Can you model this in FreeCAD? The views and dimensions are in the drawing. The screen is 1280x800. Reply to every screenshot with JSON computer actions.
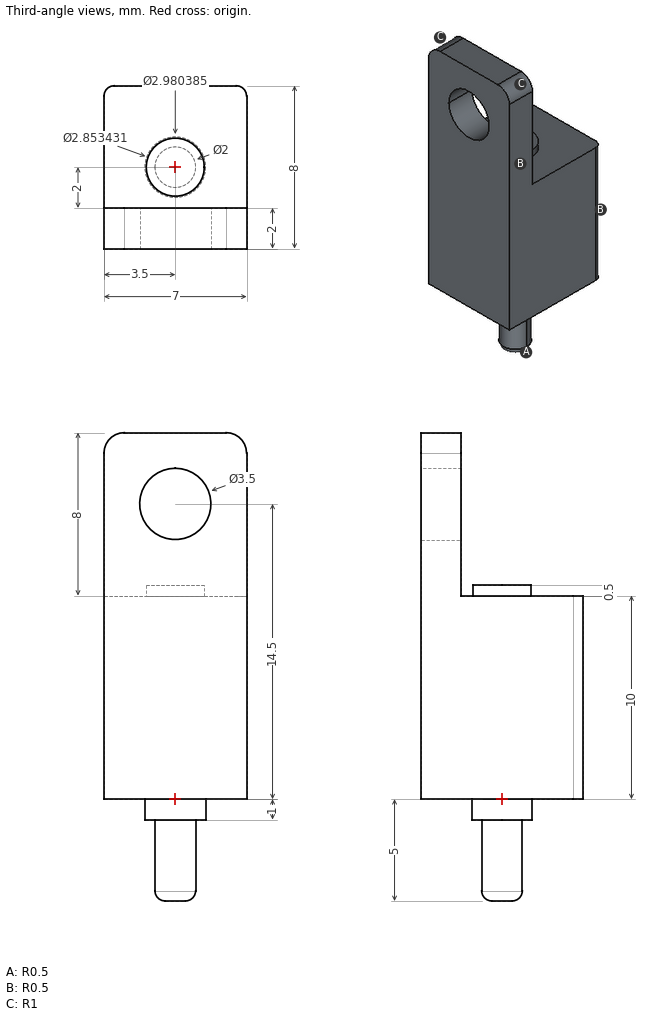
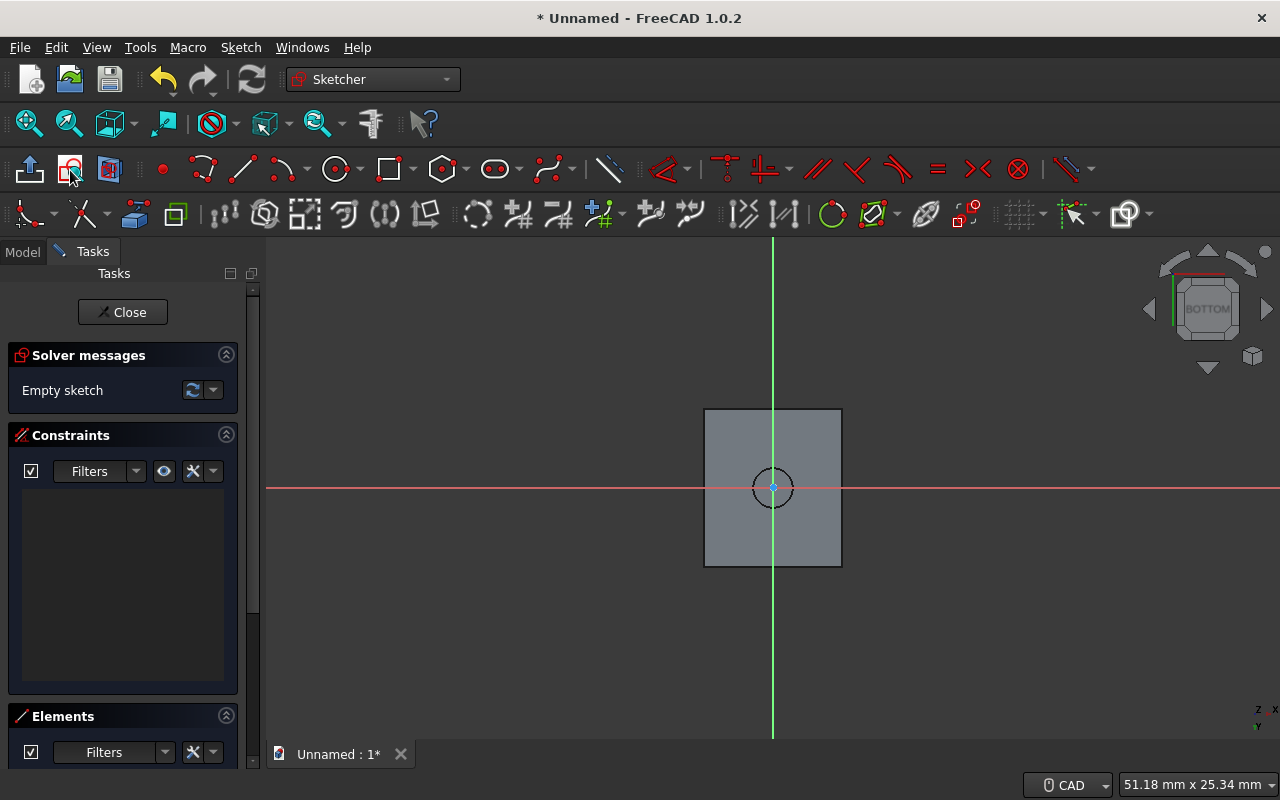
{"action": "scroll", "coordinate": [790, 488], "scroll_direction": "up", "scroll_amount": 8}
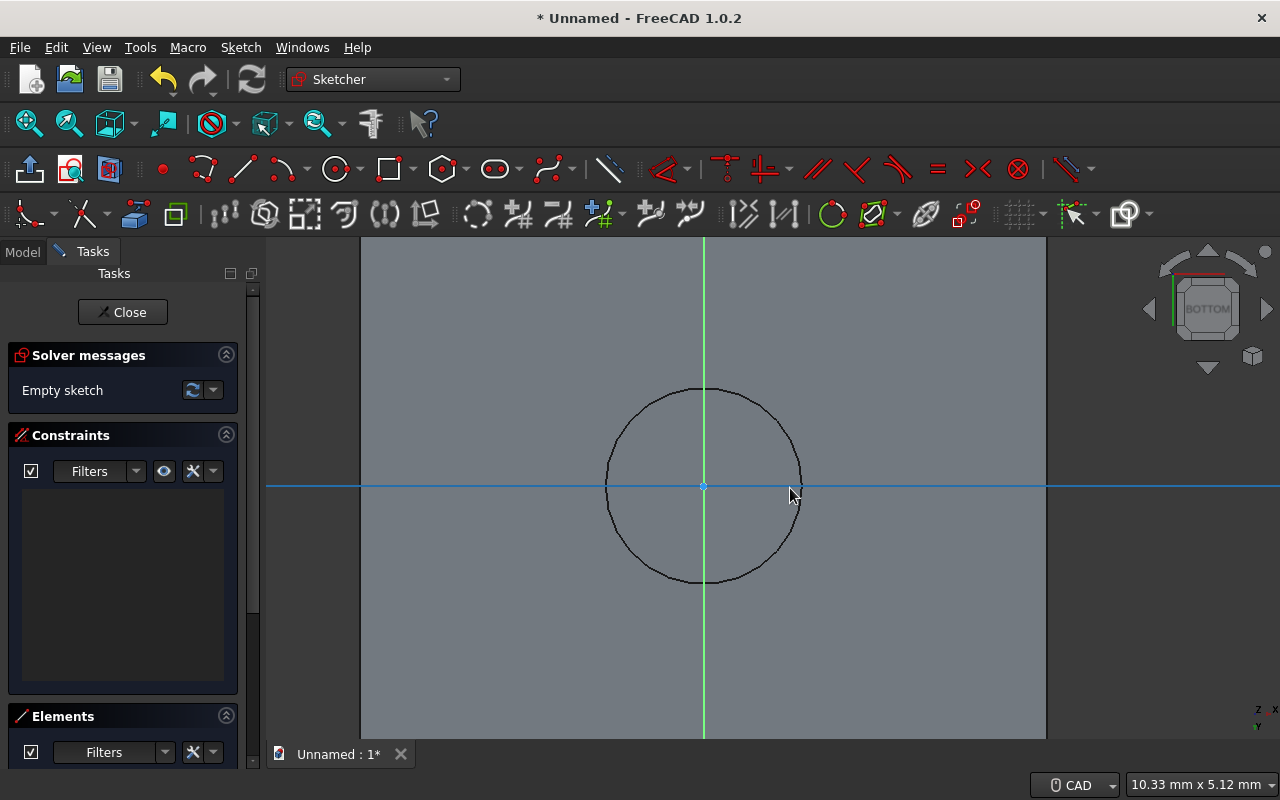
{"action": "key", "text": "g c"}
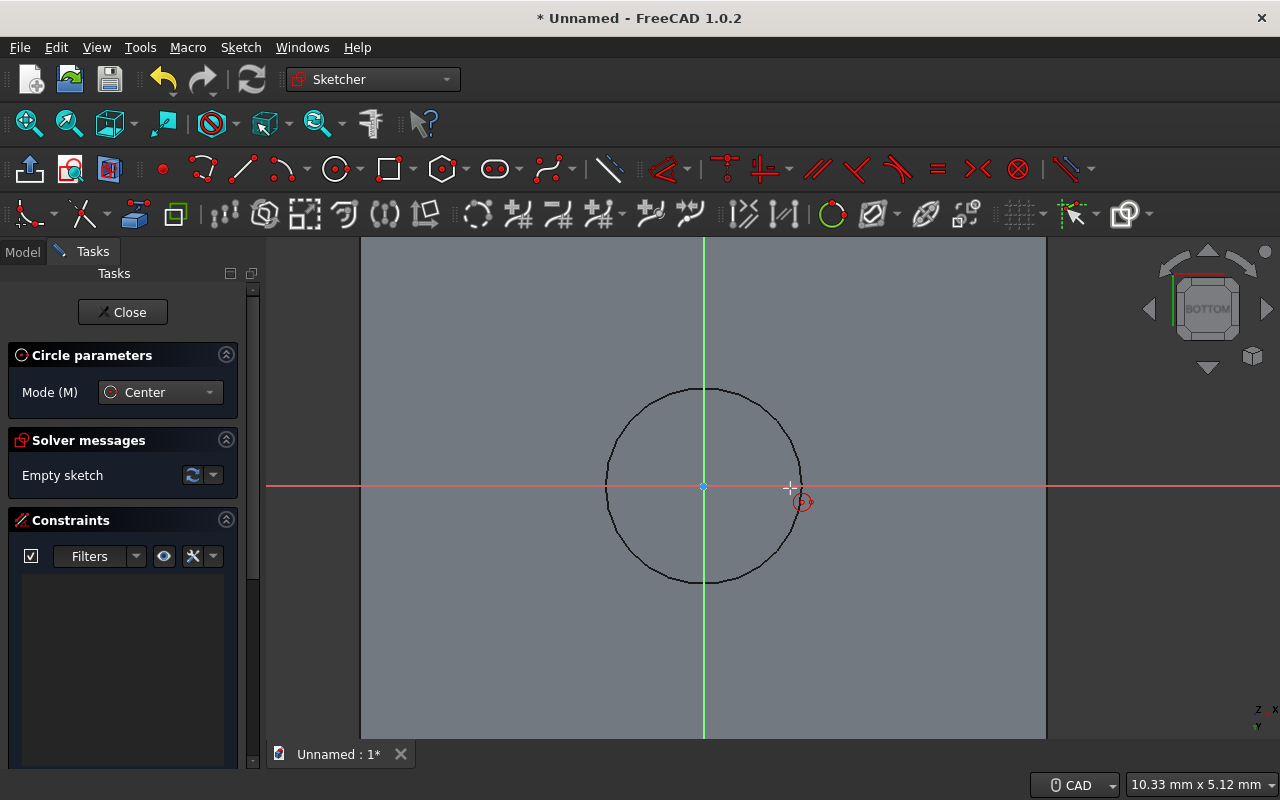
{"action": "left_click", "coordinate": [704, 486]}
{"action": "mouse_move", "coordinate": [807, 383]}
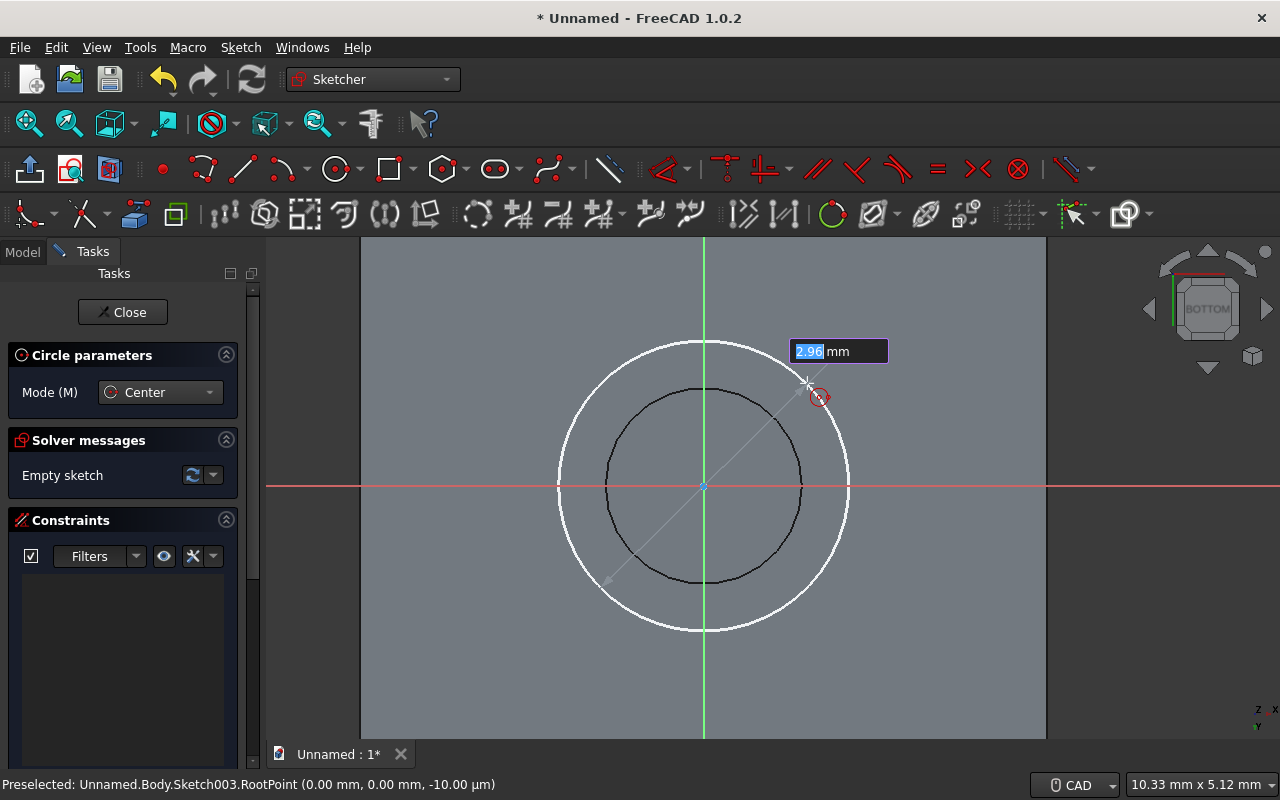
{"action": "type", "text": "2.980385"}
{"action": "key", "text": "Return"}
{"action": "key", "text": "Escape"}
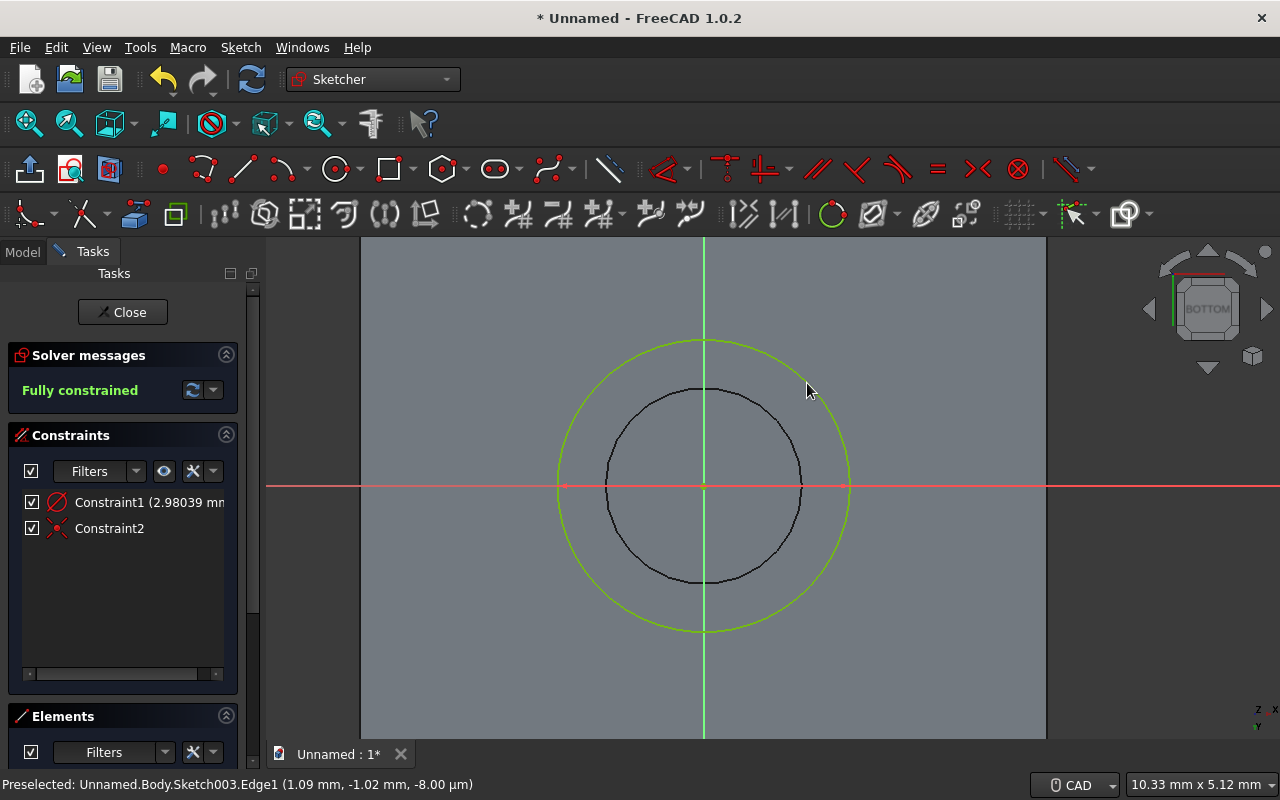
{"action": "left_click", "coordinate": [123, 312]}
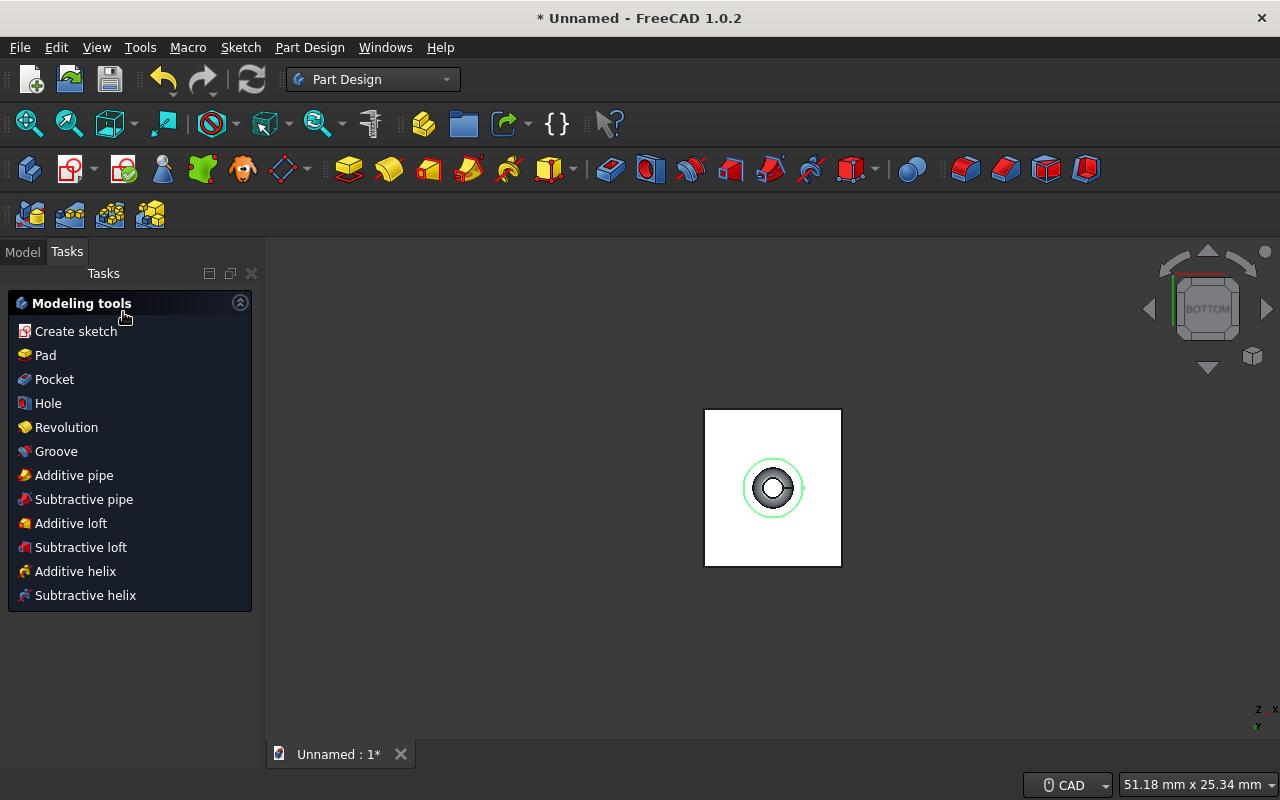
{"action": "left_click", "coordinate": [350, 170]}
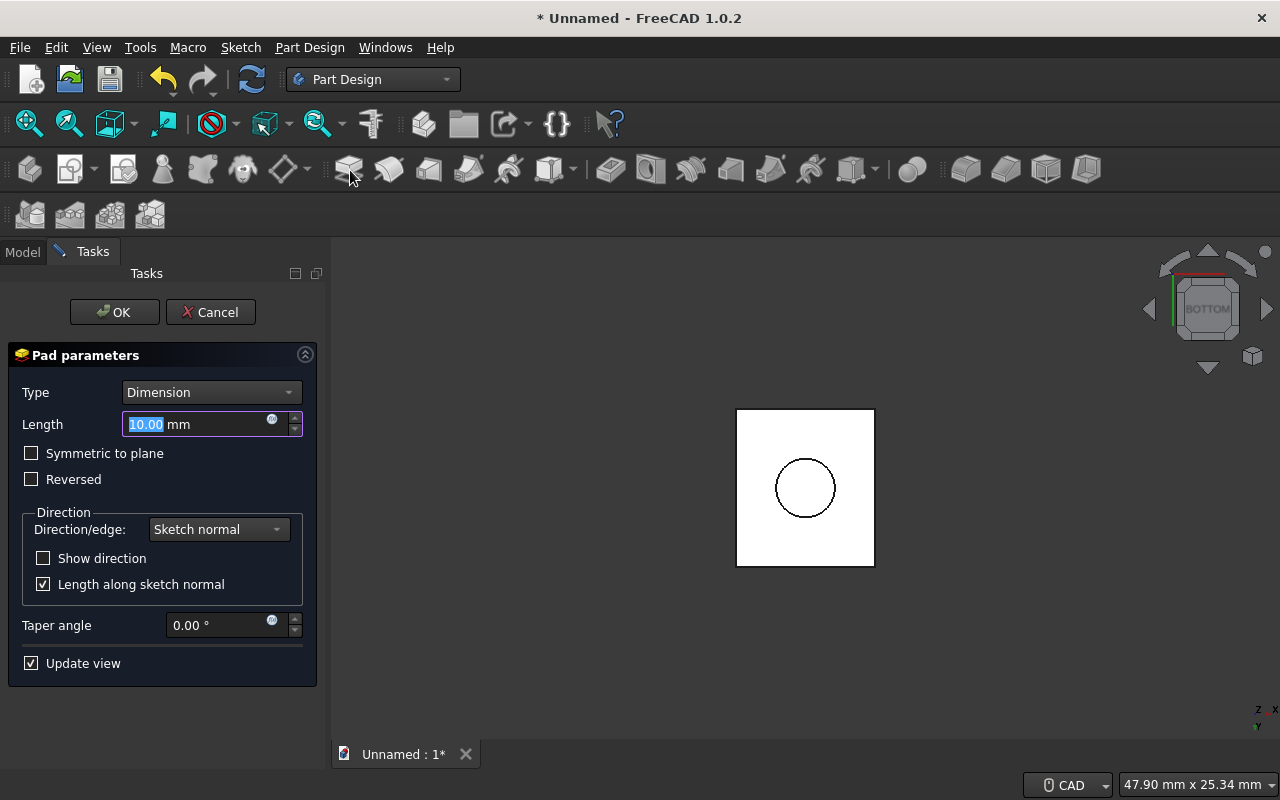
{"action": "type", "text": "1"}
{"action": "key", "text": "Tab"}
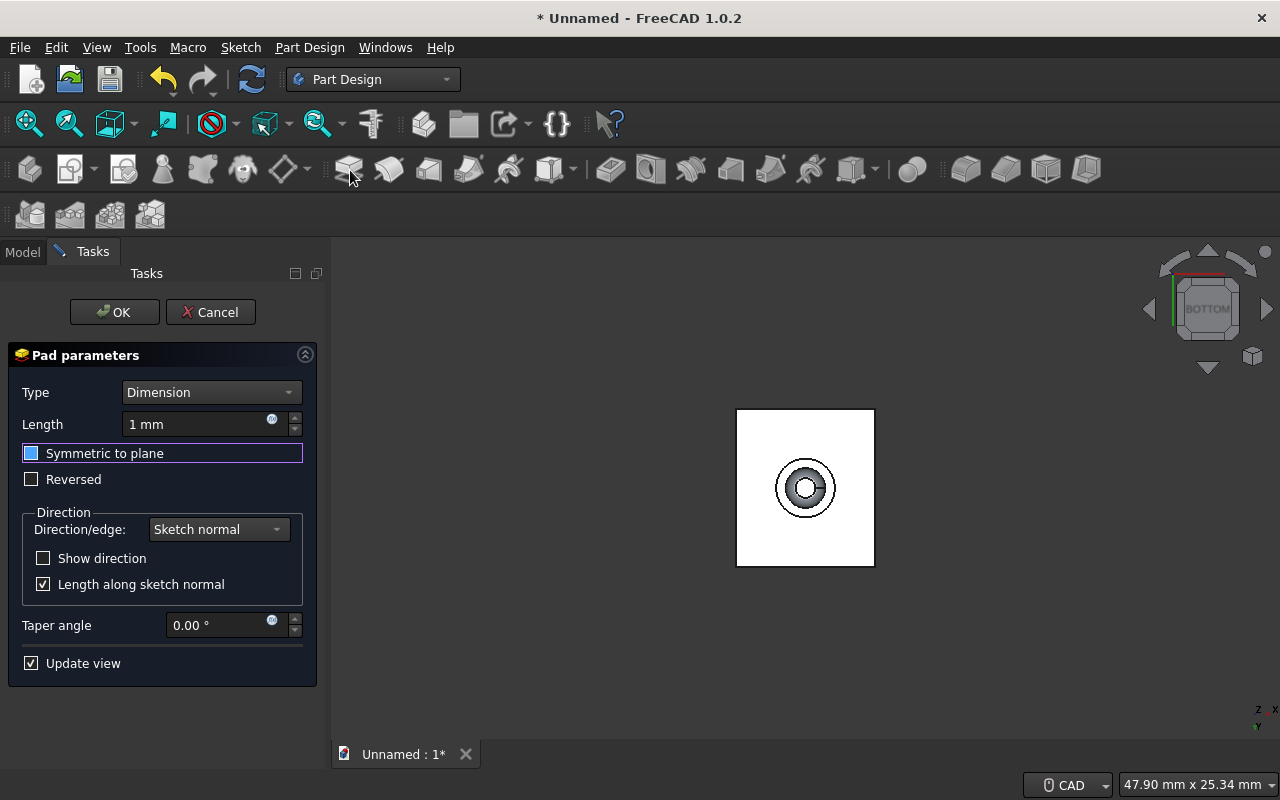
{"action": "left_click", "coordinate": [115, 312]}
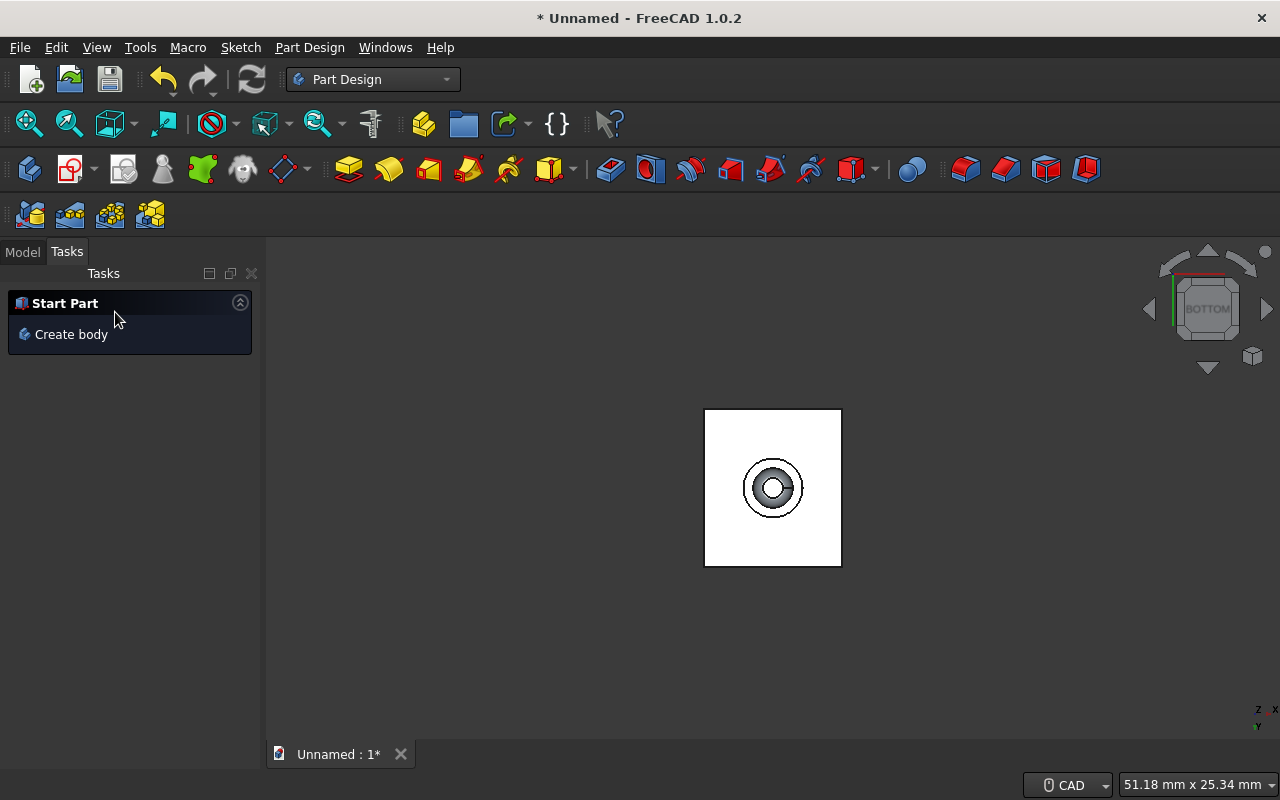
{"action": "left_click", "coordinate": [30, 124]}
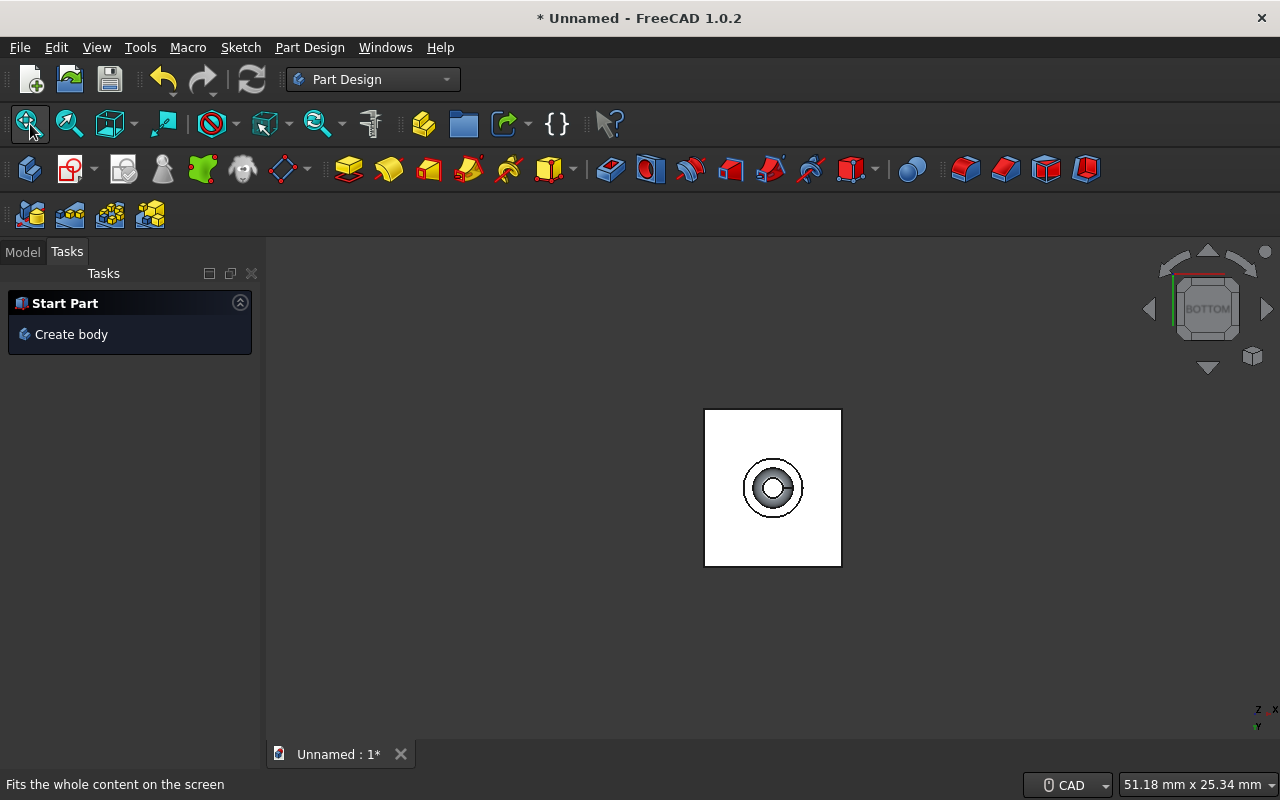
{"action": "key", "text": "0"}